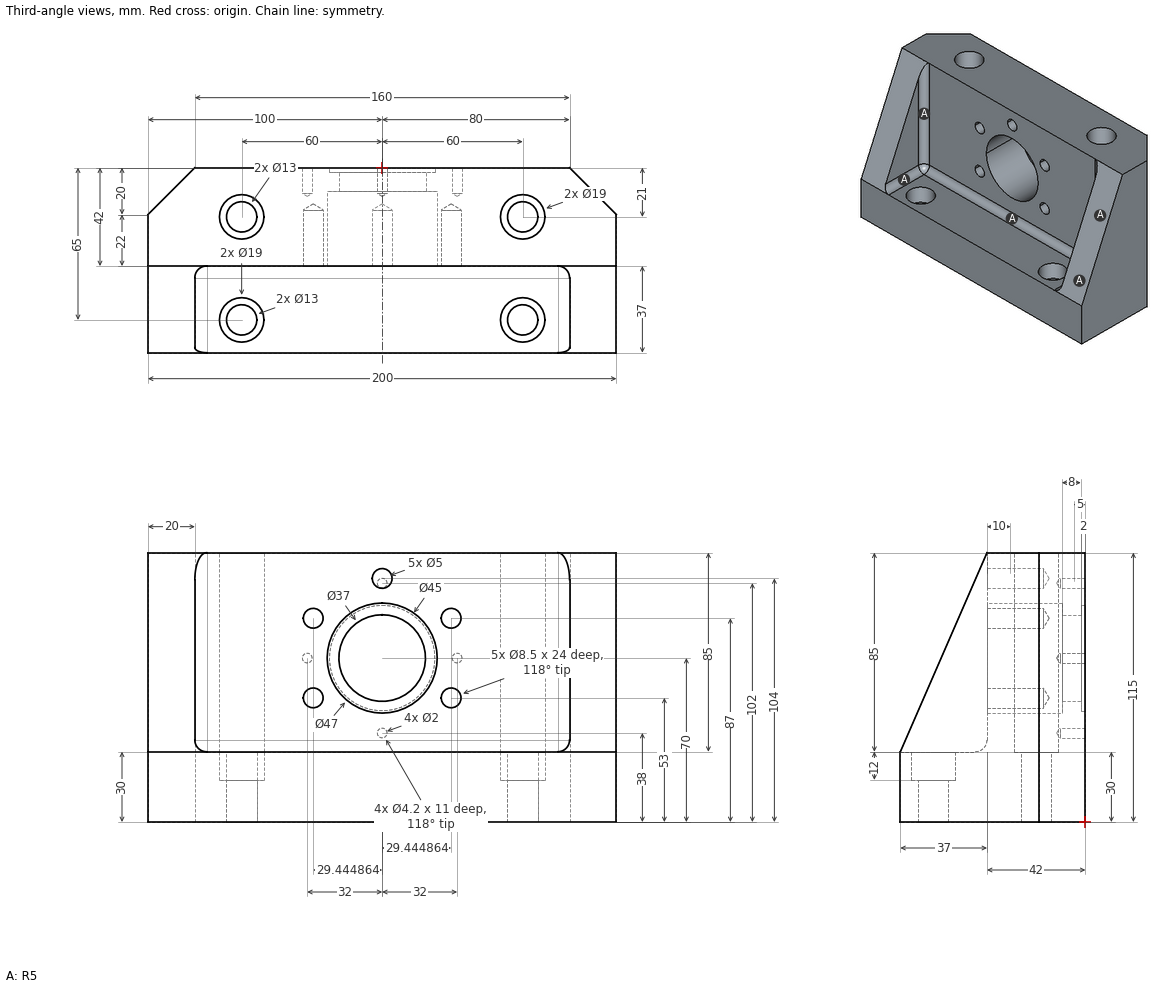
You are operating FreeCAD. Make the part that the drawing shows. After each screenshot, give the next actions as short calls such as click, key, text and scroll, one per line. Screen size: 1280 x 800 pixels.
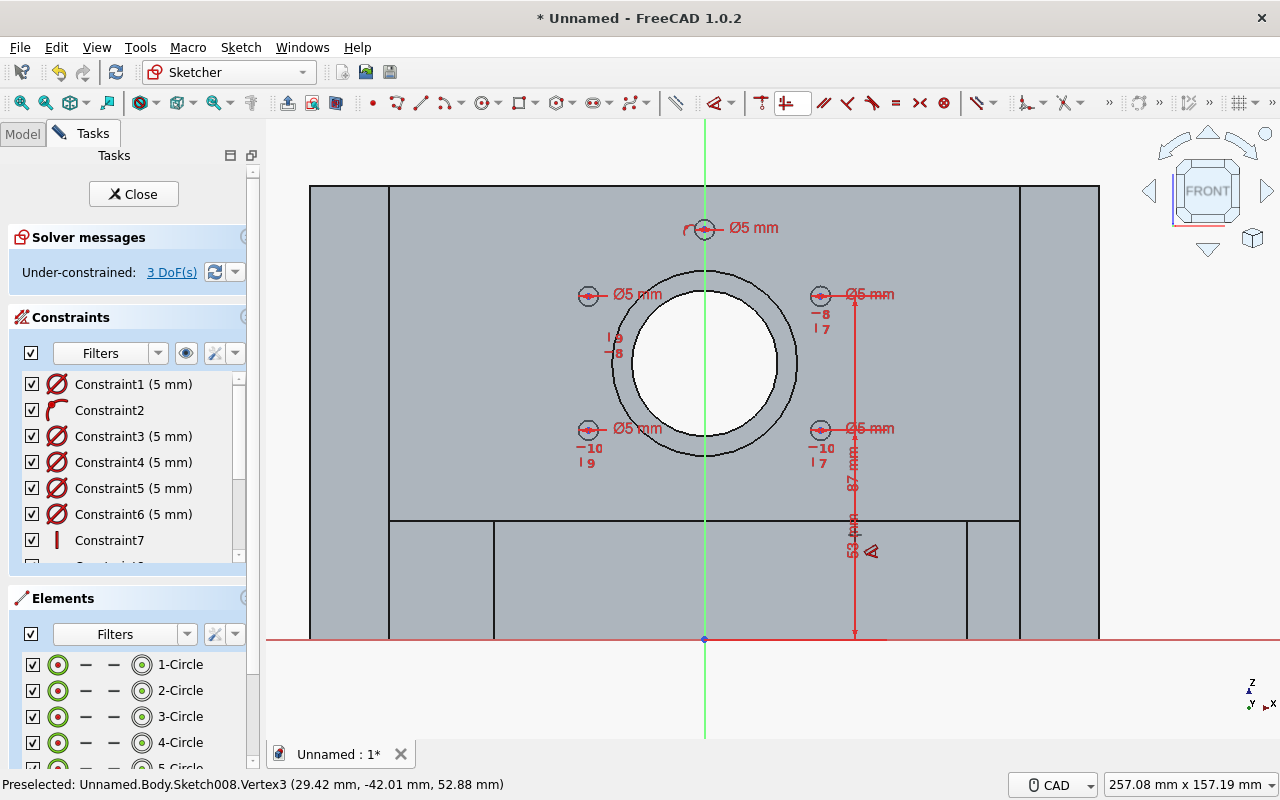
click(705, 230)
click(739, 435)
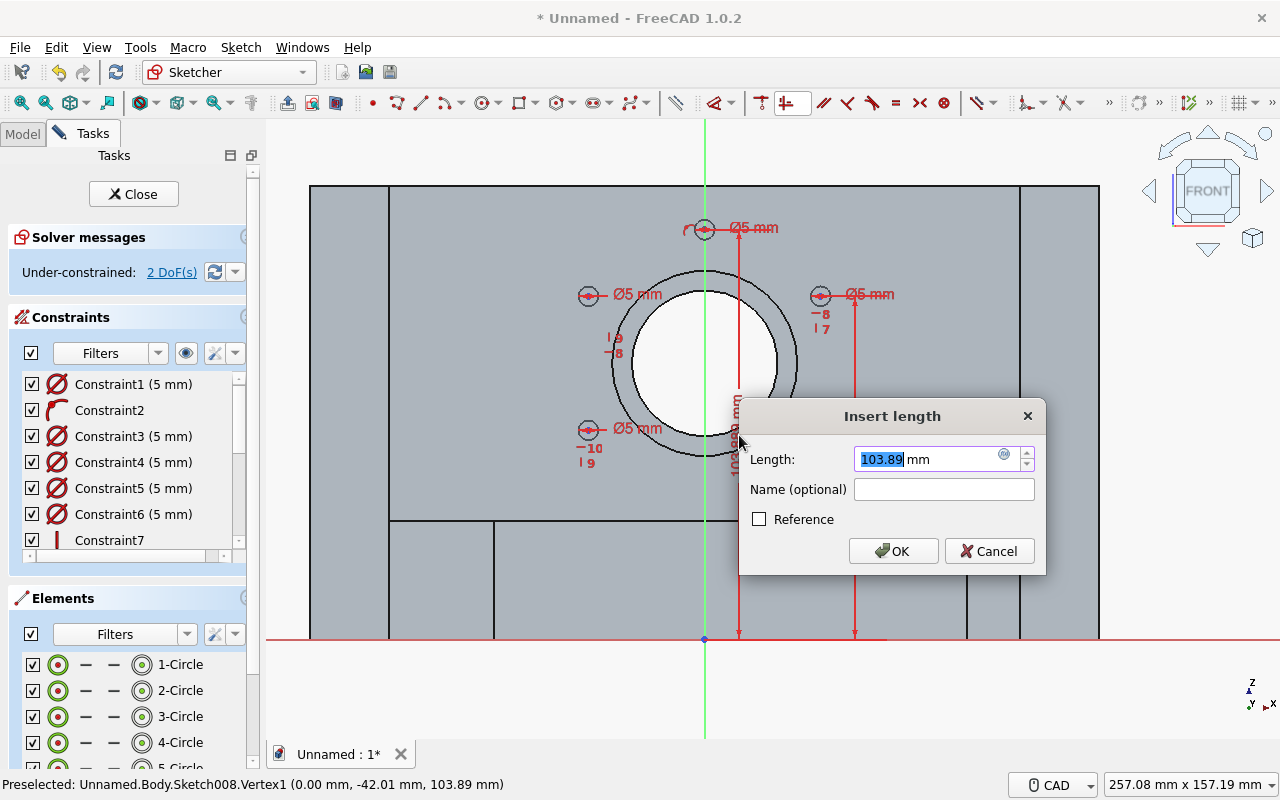
text(104)
key(Return)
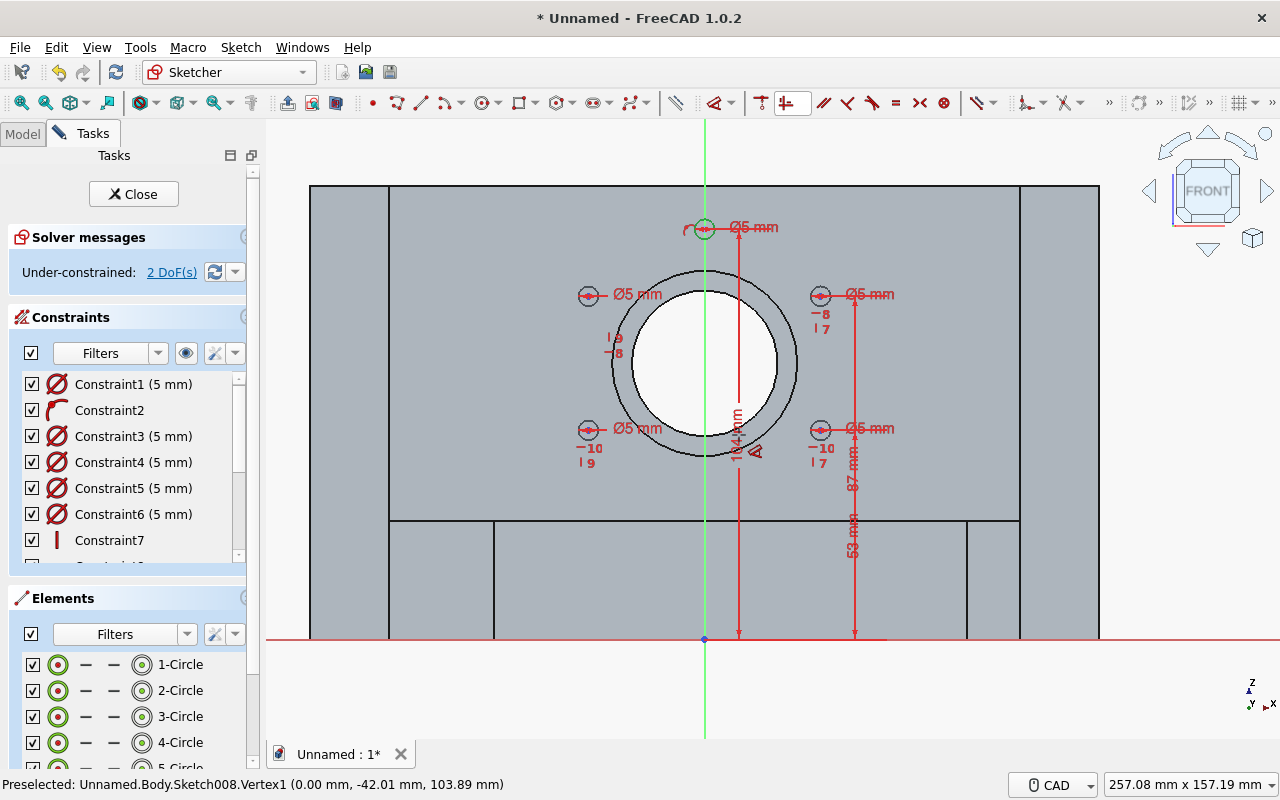
click(821, 296)
click(763, 674)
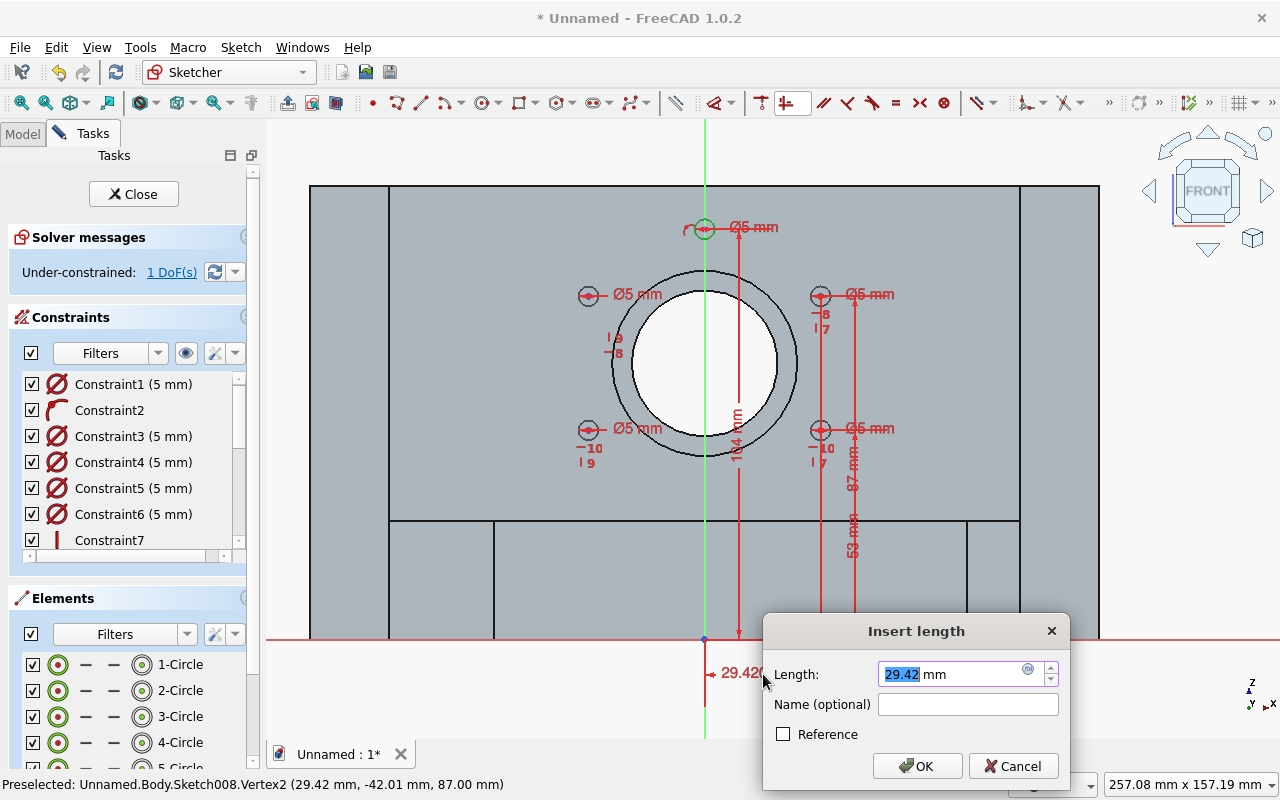
text(29.444864)
key(Return)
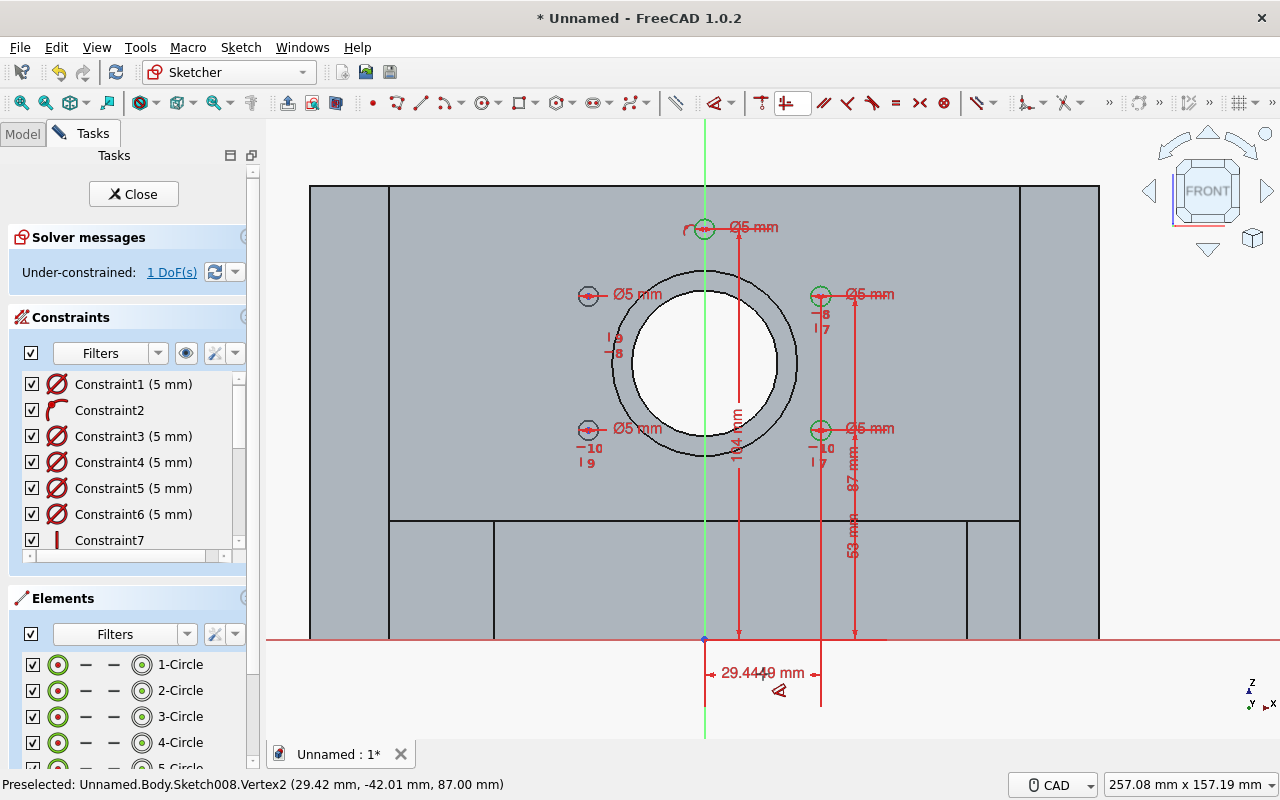
click(588, 296)
click(647, 674)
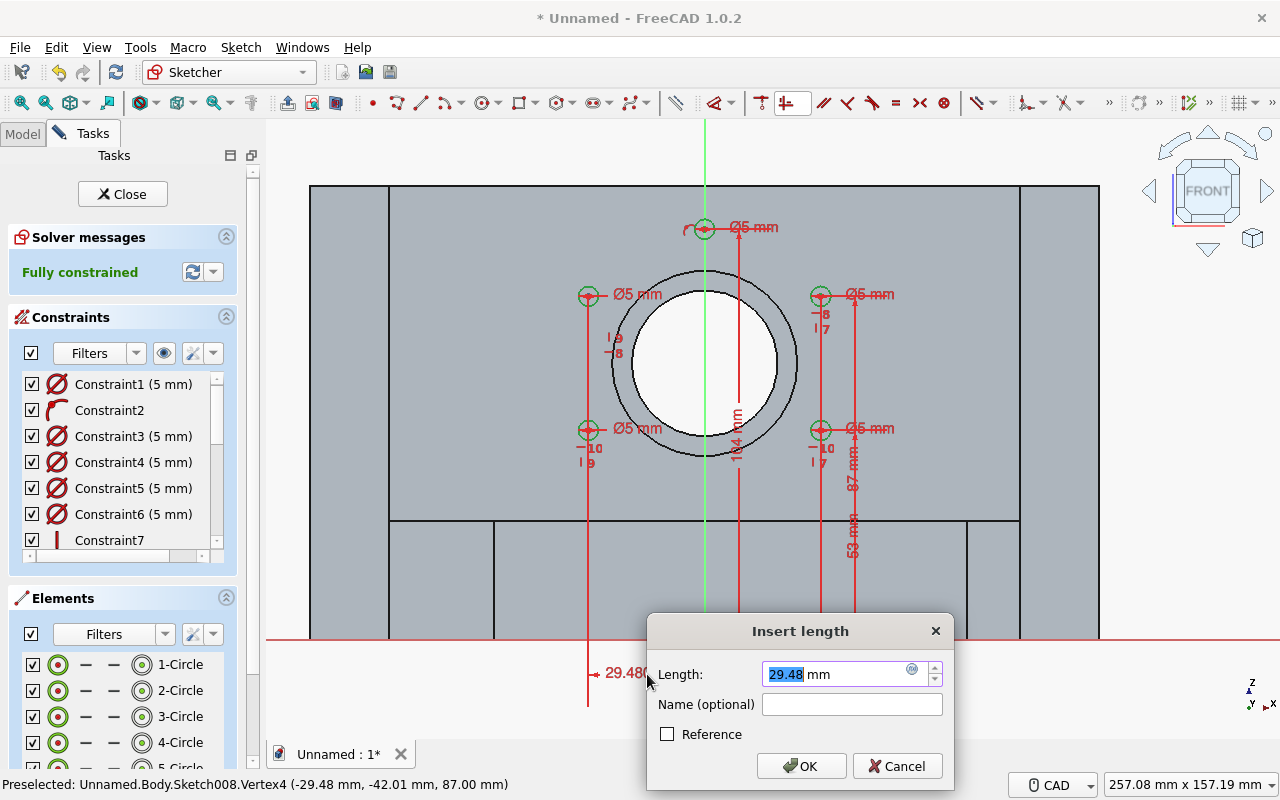
text(29.444864)
key(Return)
key(Escape)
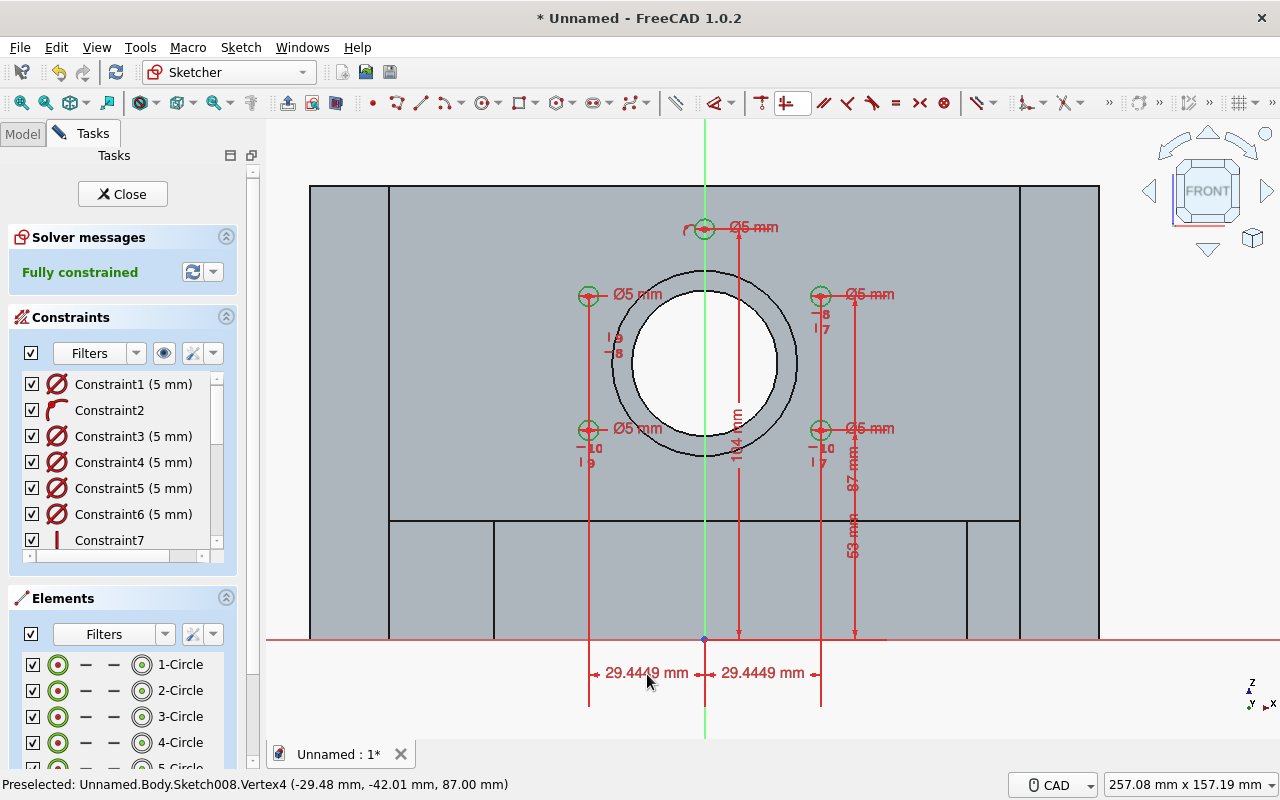
click(123, 194)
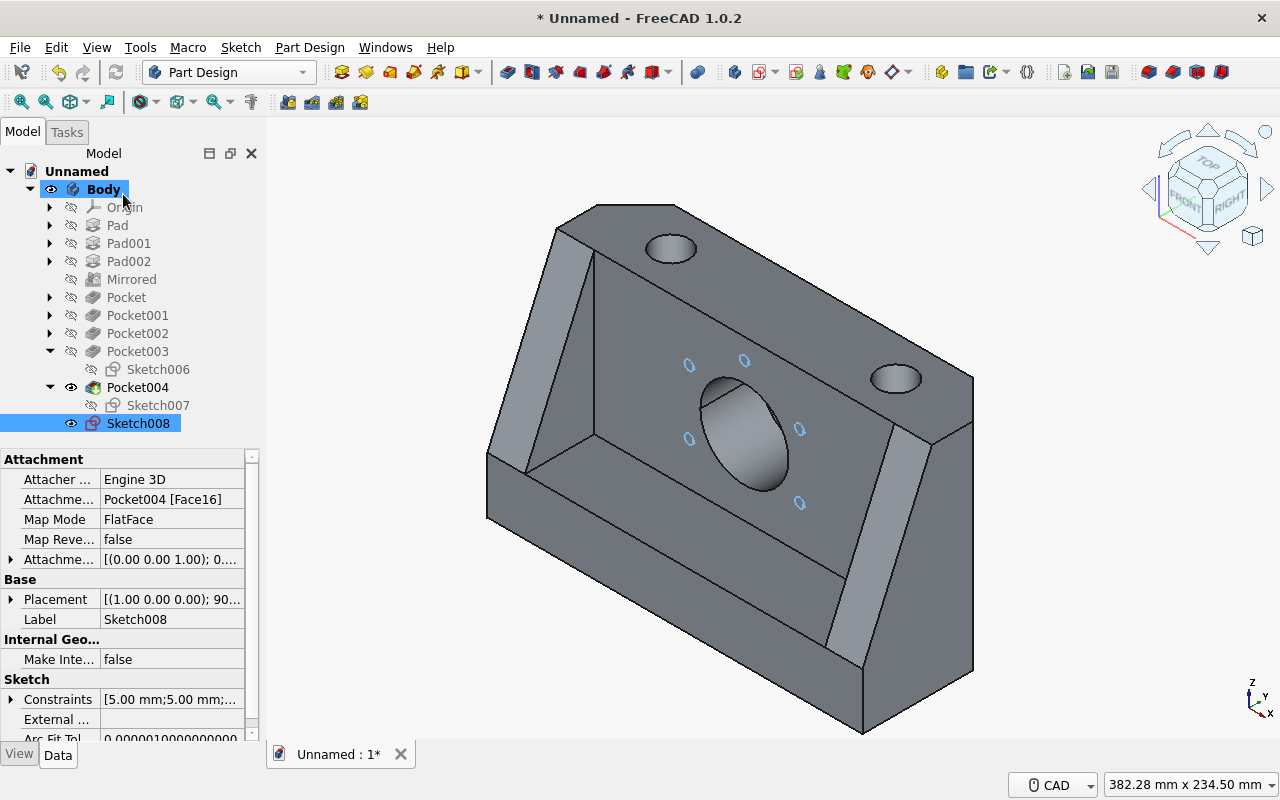
click(508, 72)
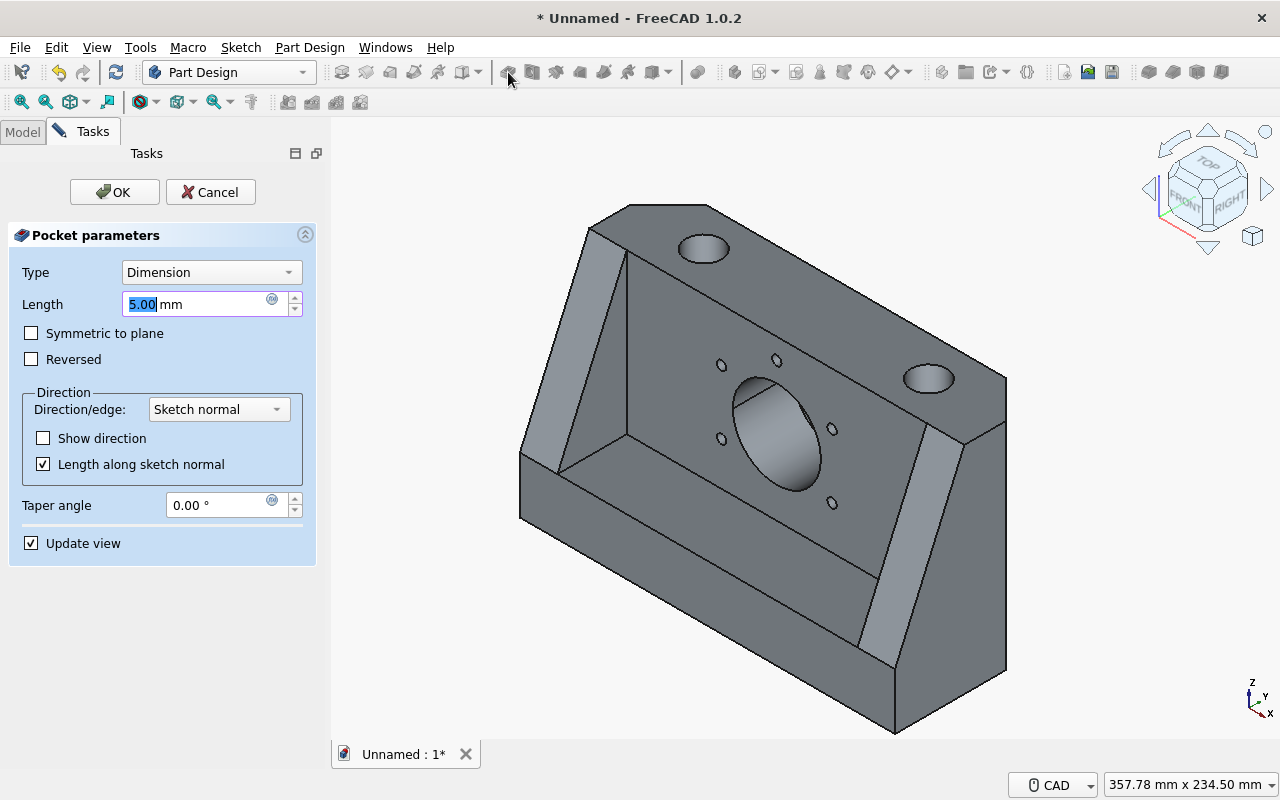
text(10)
key(Tab)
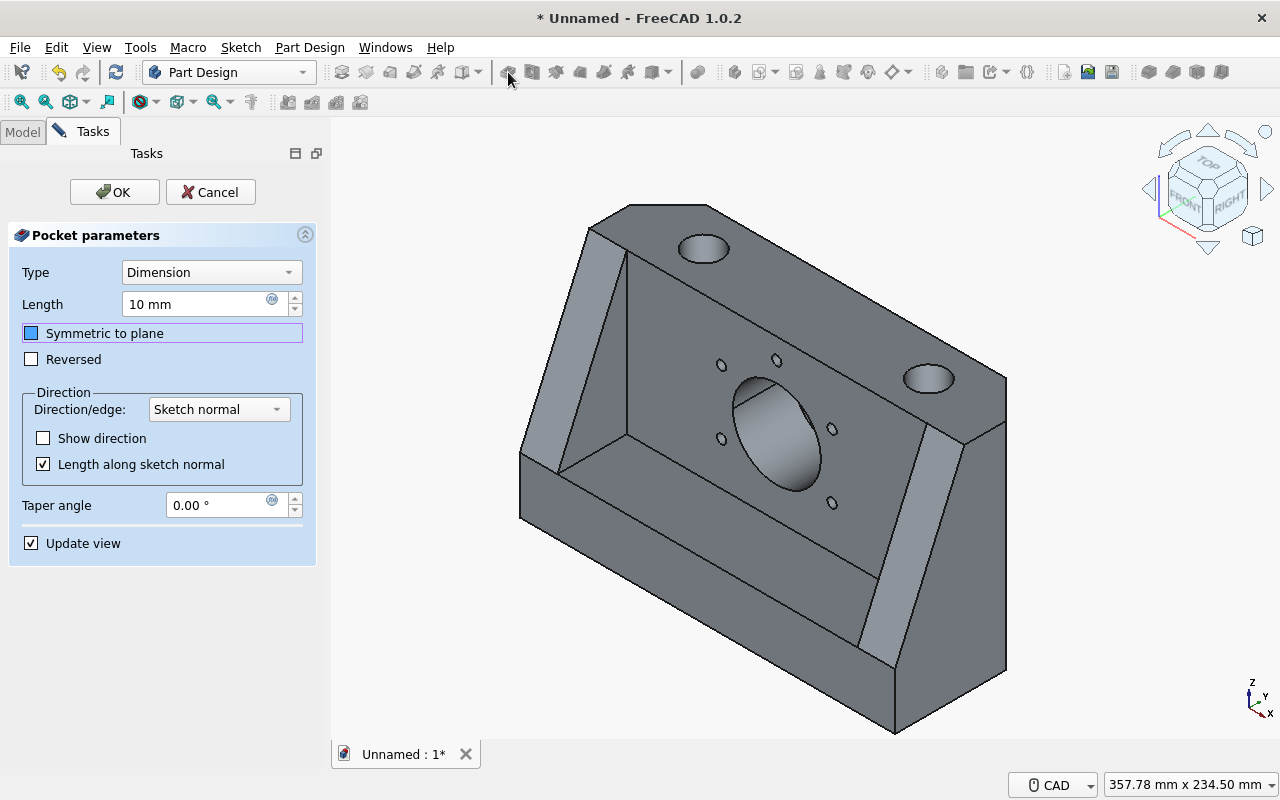
click(115, 192)